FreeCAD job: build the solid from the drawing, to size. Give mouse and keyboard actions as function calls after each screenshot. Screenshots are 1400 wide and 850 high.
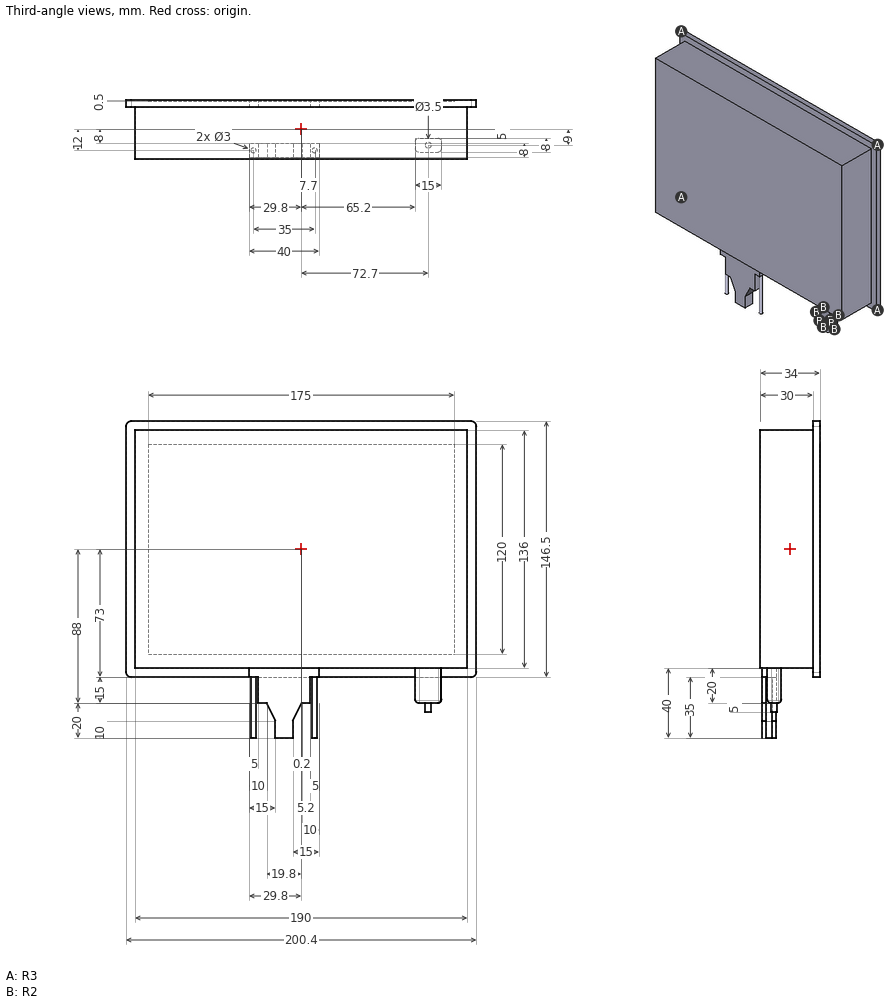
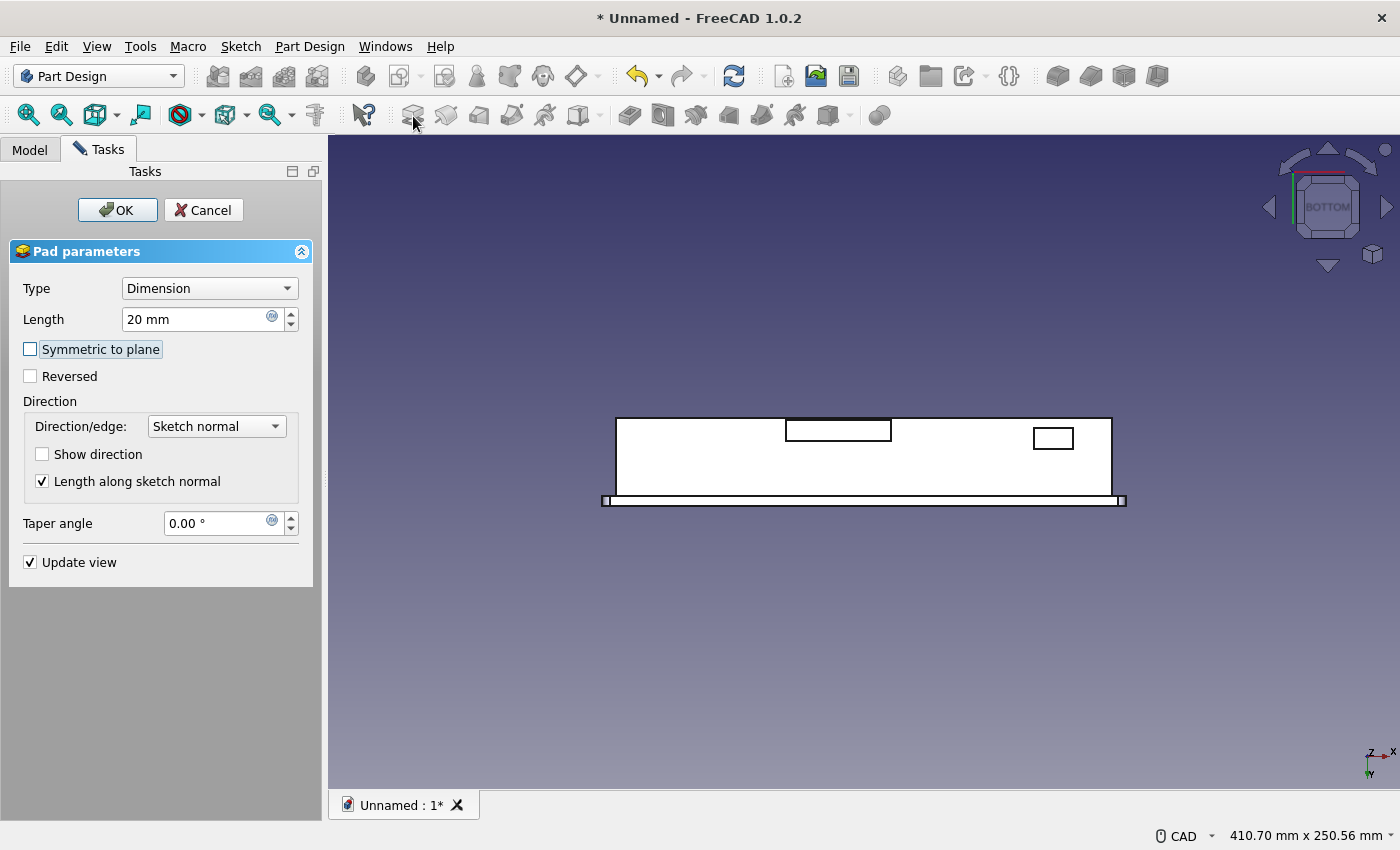
click(118, 210)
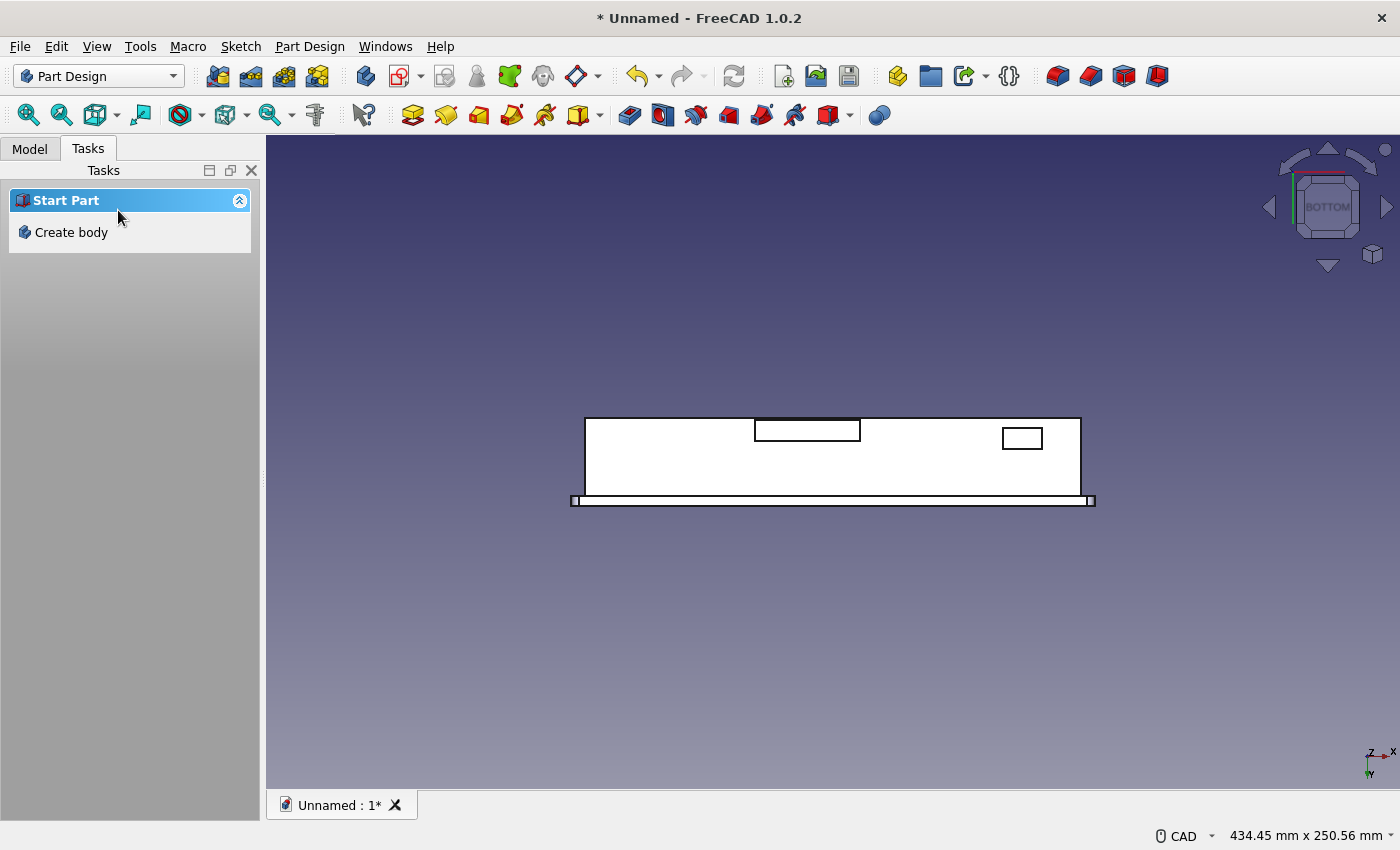
click(1028, 438)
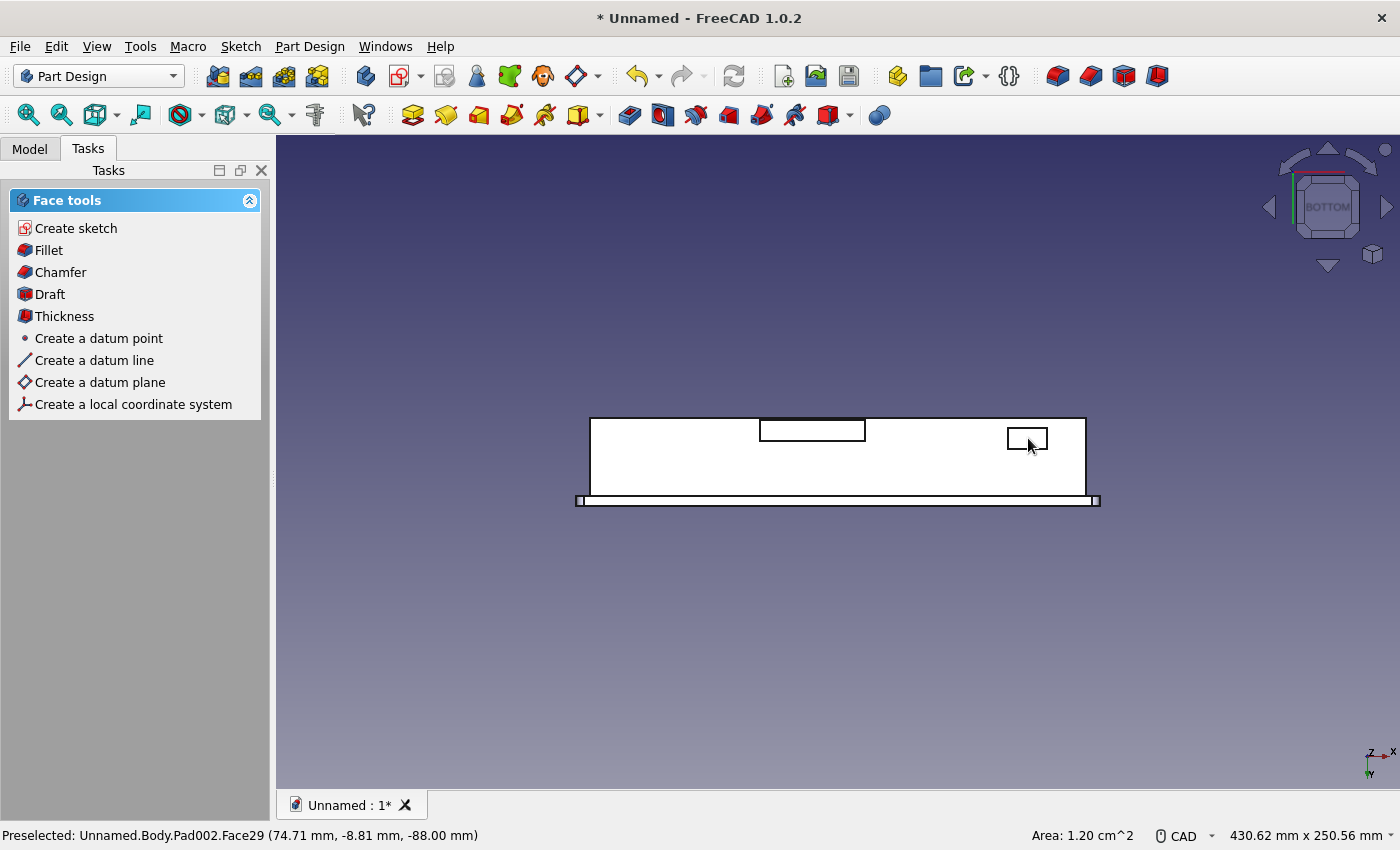
key(0)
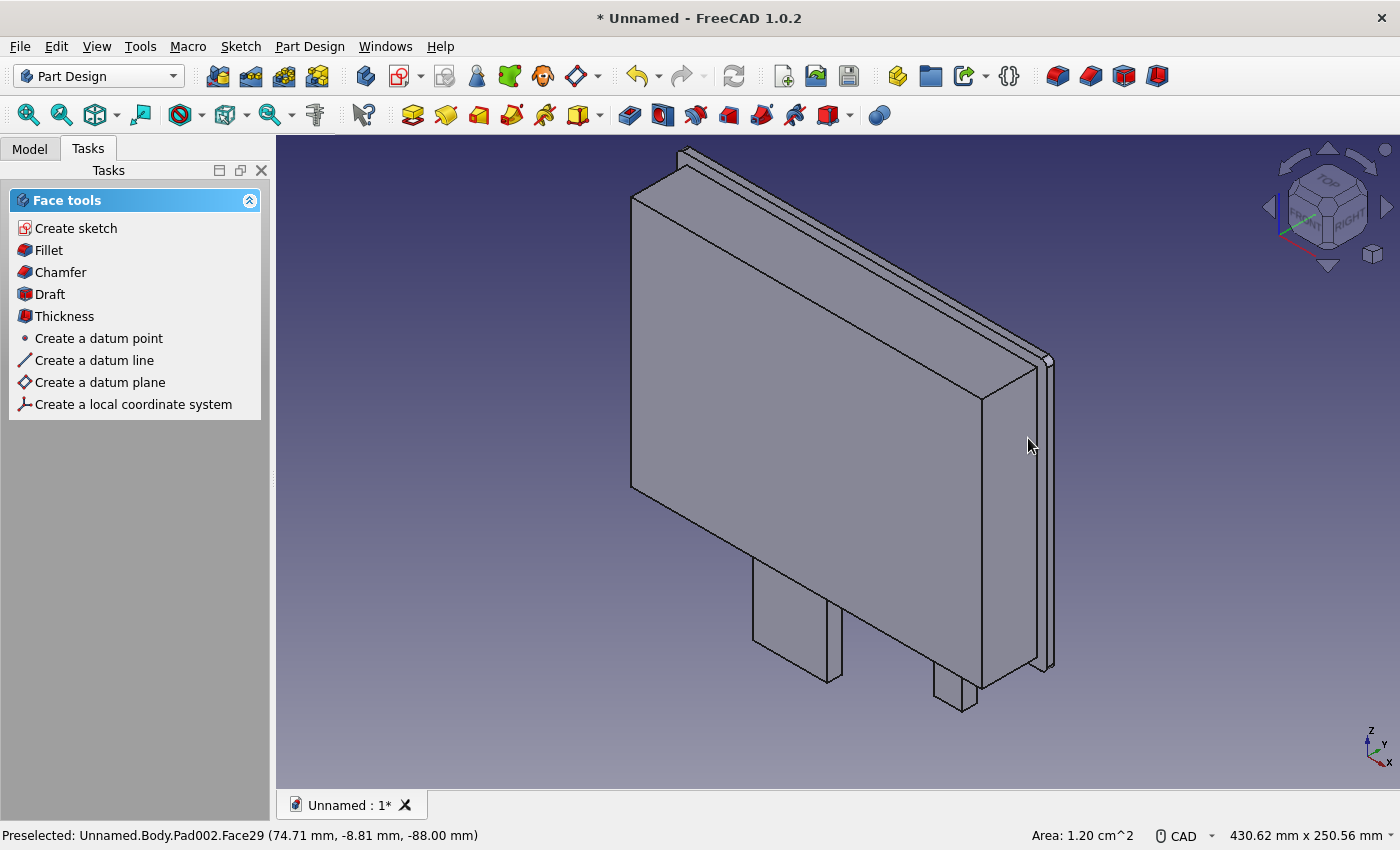
click(962, 690, ctrl)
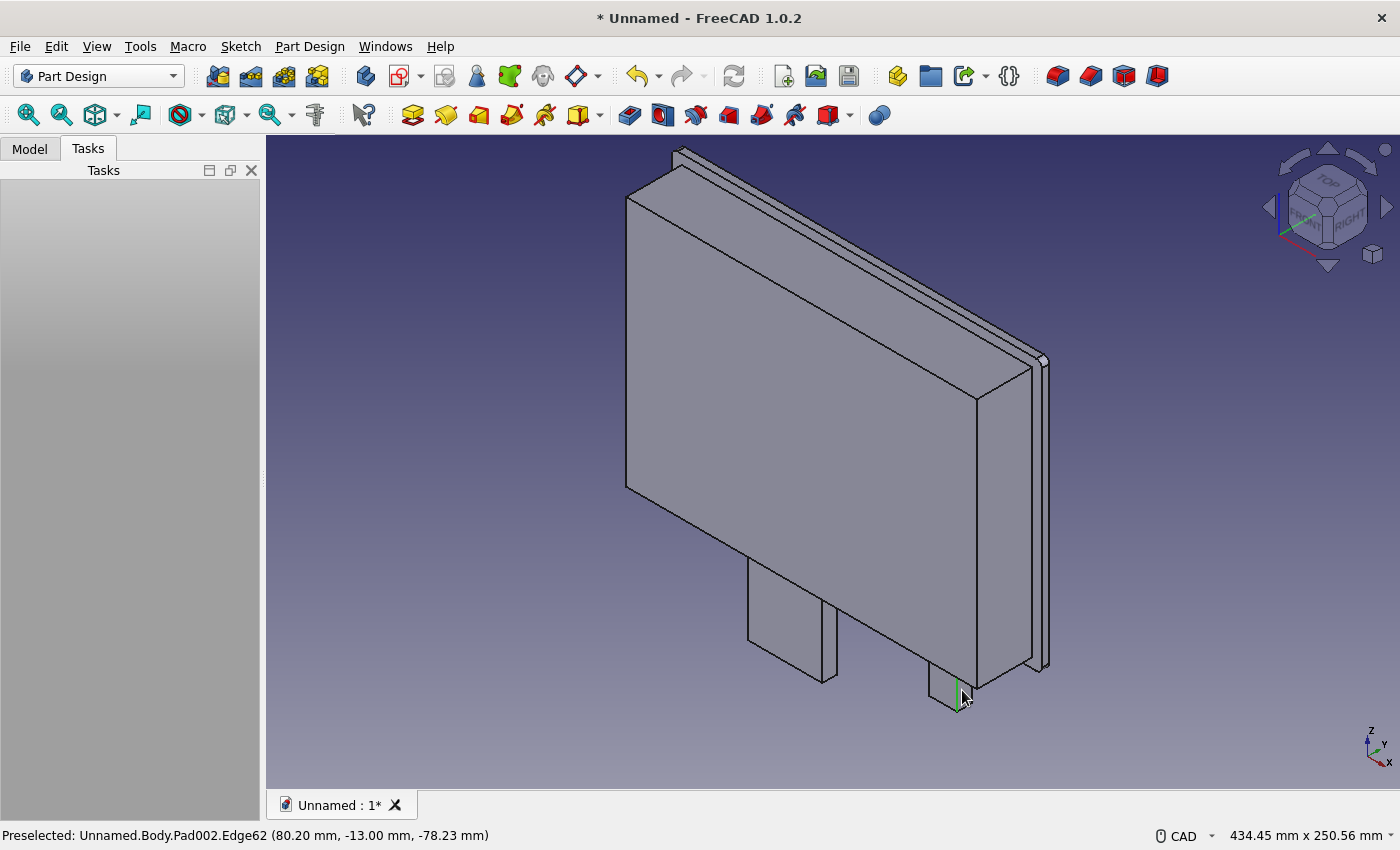
key(2)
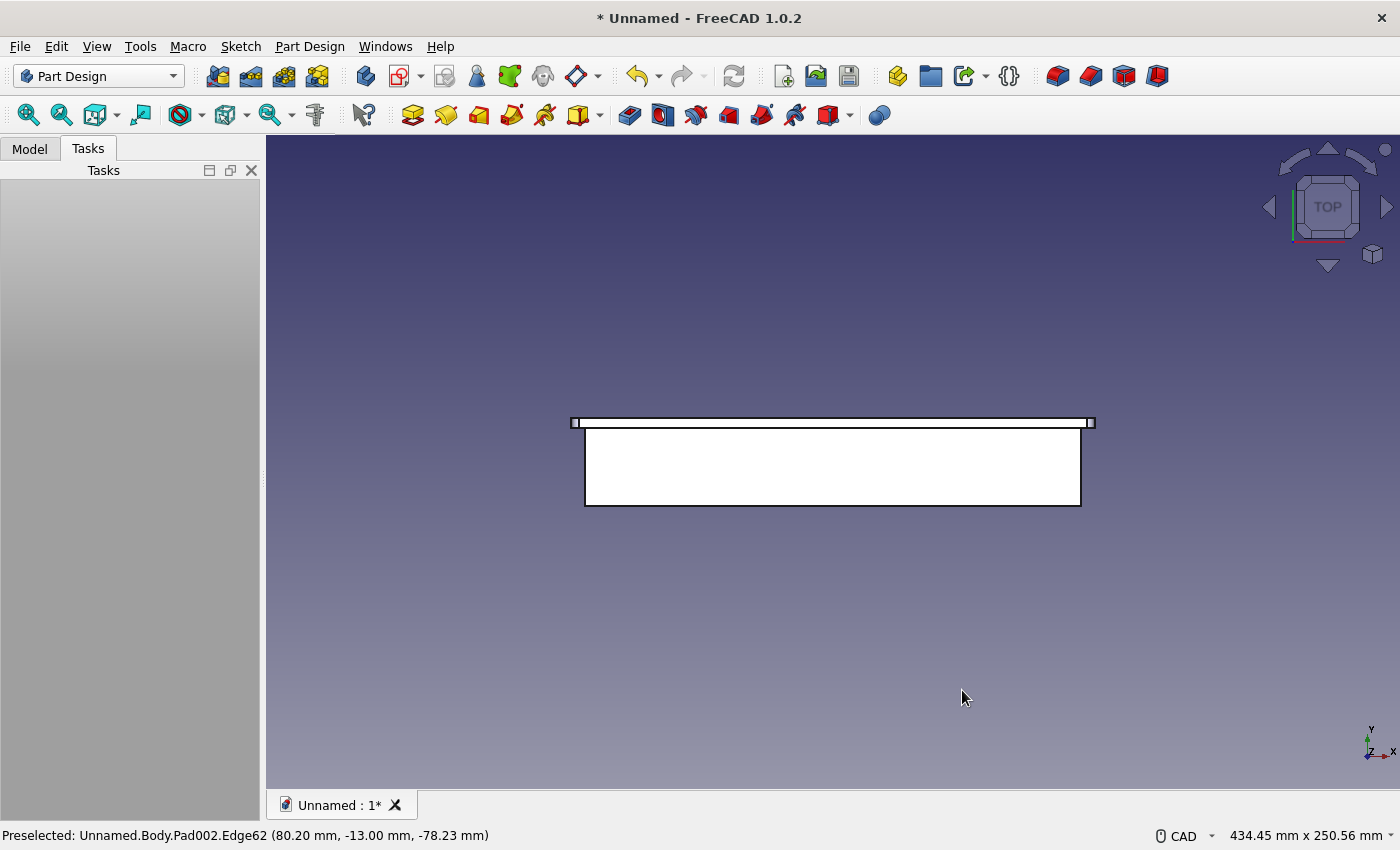
key(1)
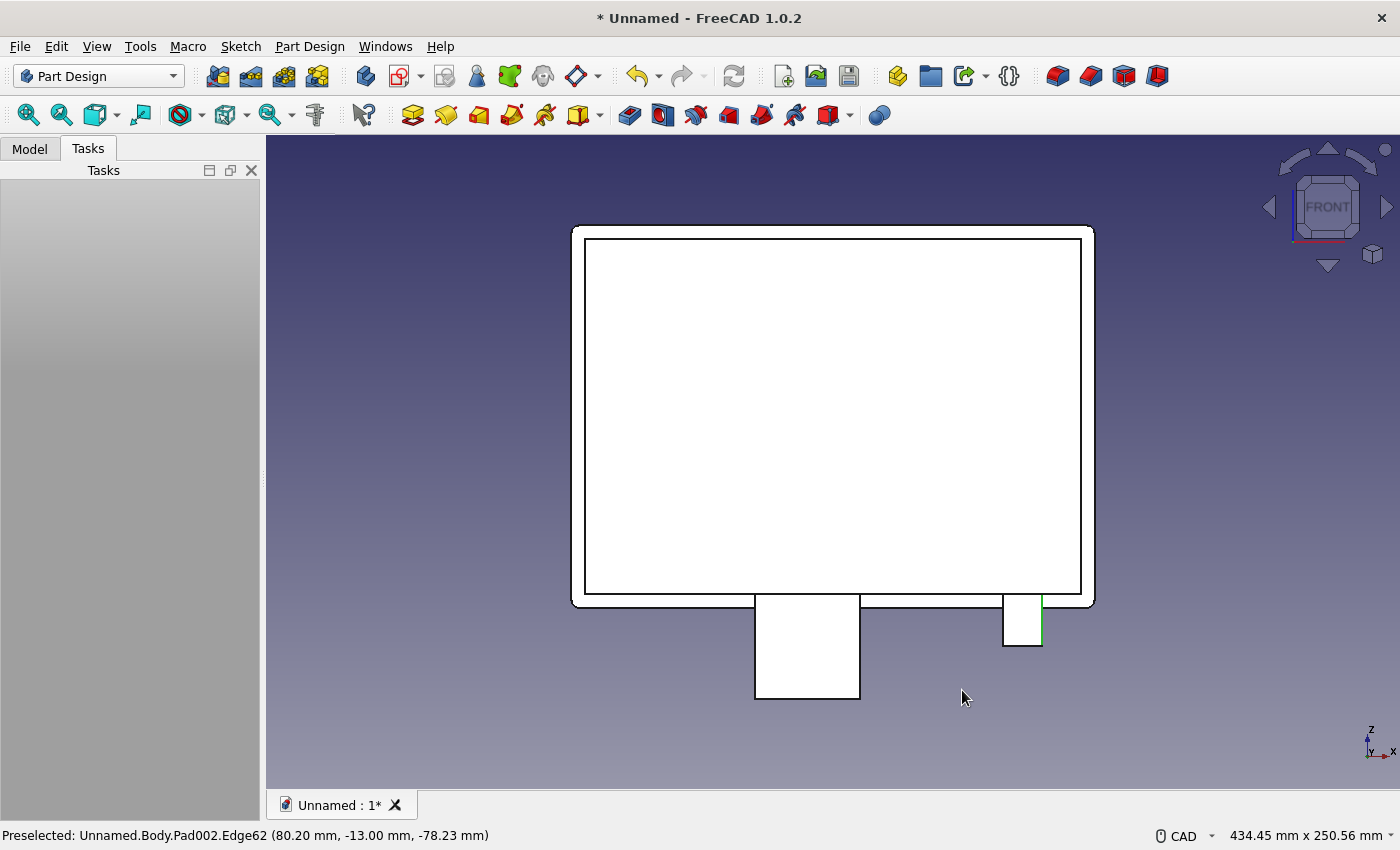
click(1003, 619, ctrl)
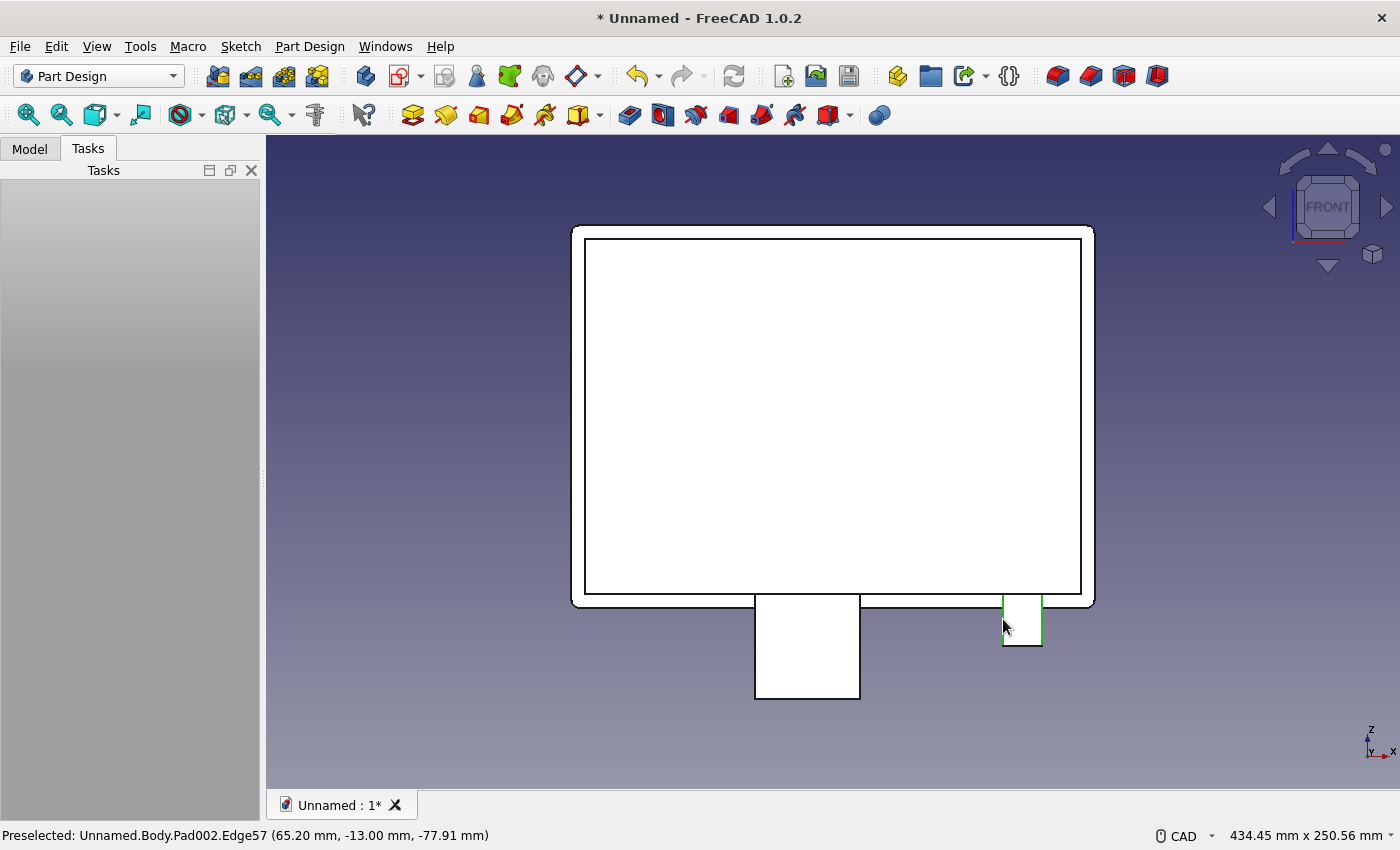
key(3)